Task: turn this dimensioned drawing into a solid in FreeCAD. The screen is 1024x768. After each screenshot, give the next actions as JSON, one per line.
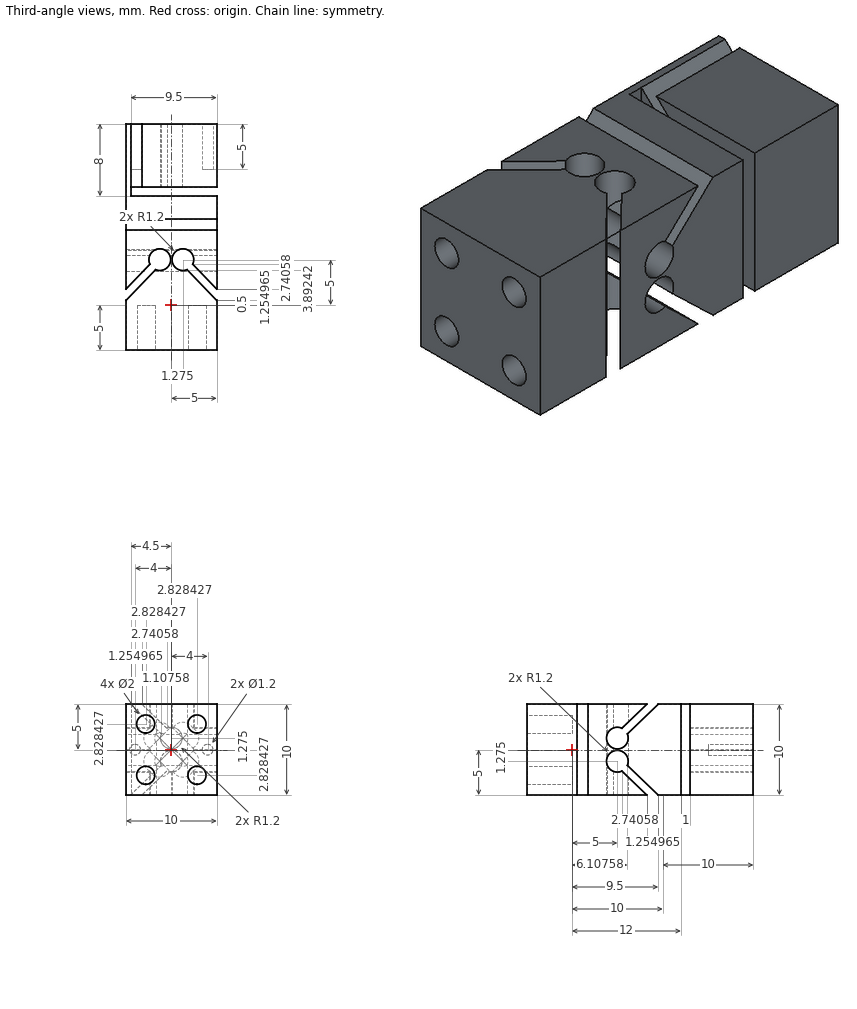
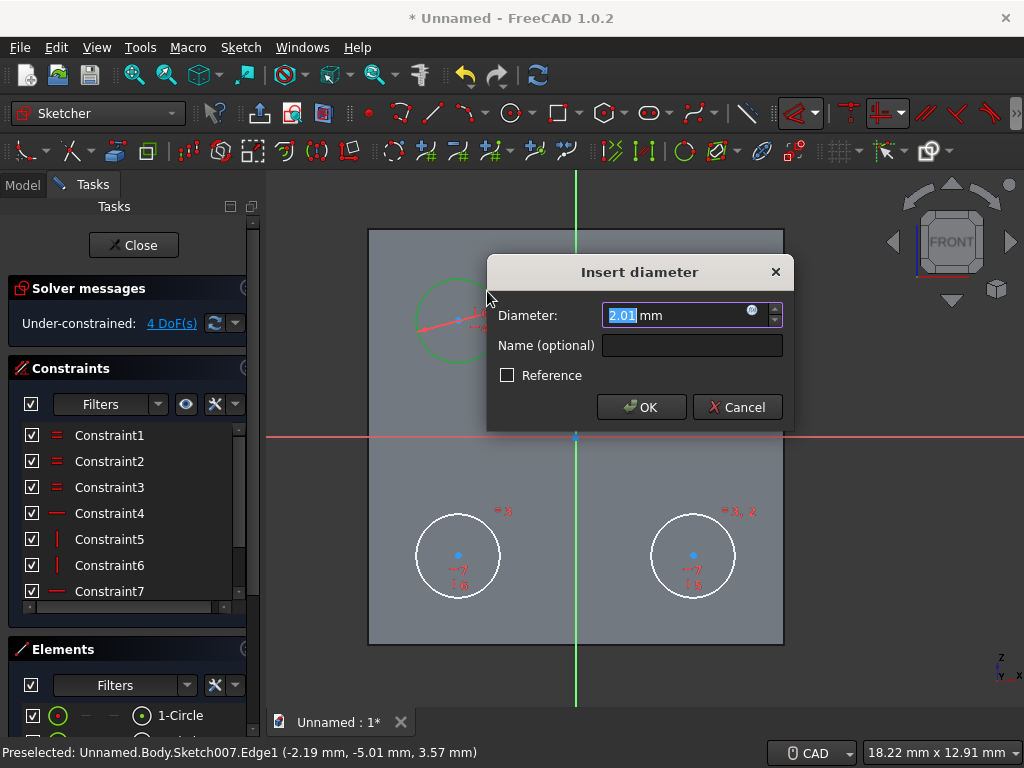
{"action": "type", "text": "2"}
{"action": "key", "text": "Return"}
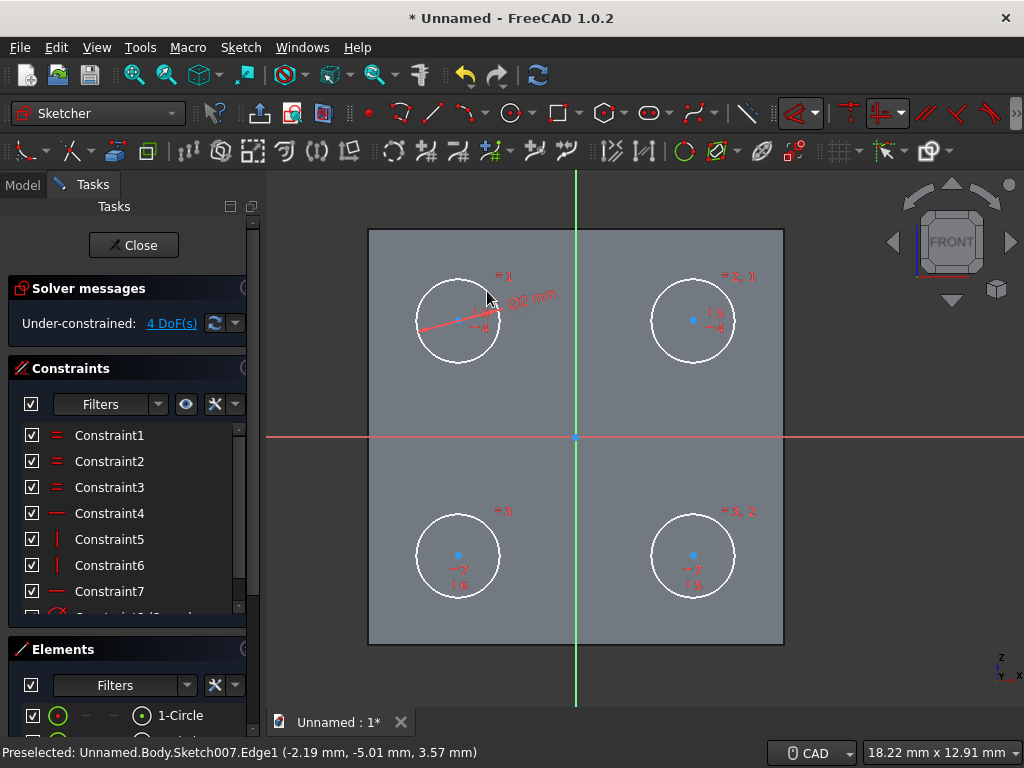
{"action": "left_click", "coordinate": [458, 321]}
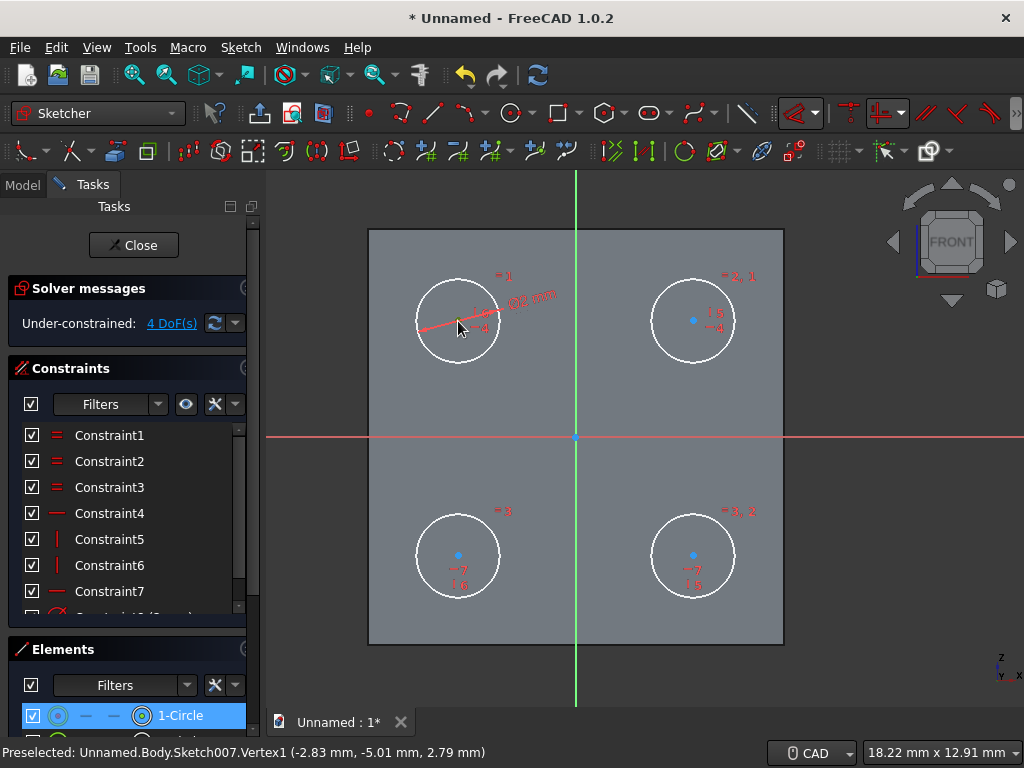
{"action": "key", "text": "l"}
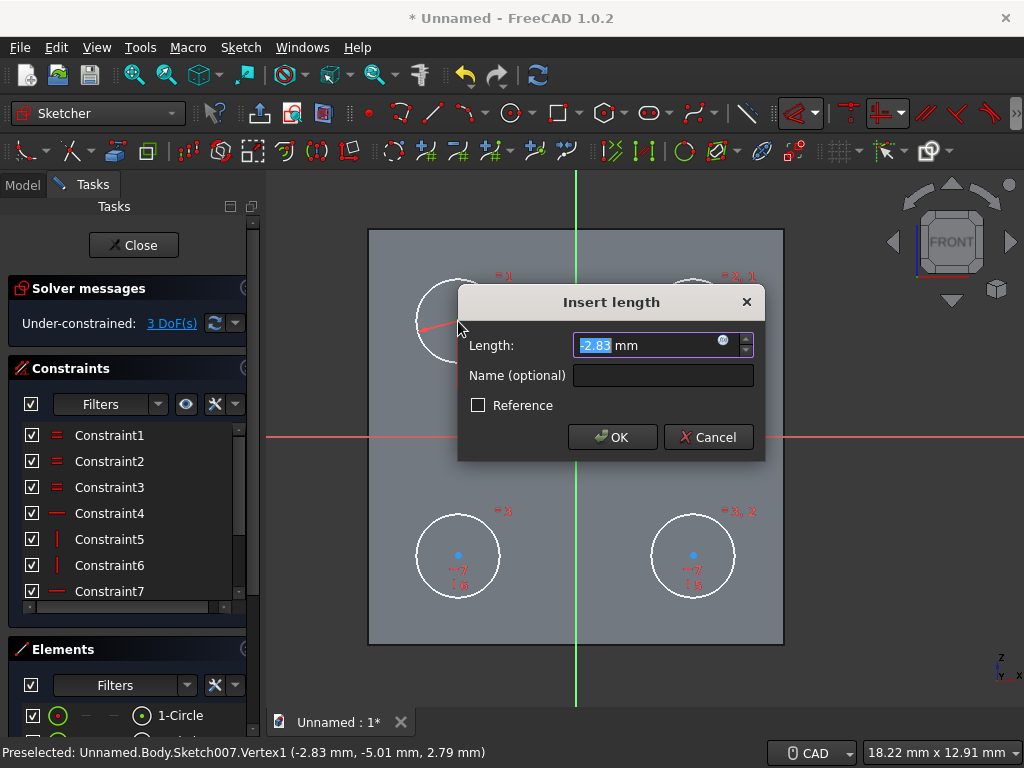
{"action": "type", "text": "-2.828427"}
{"action": "key", "text": "Return"}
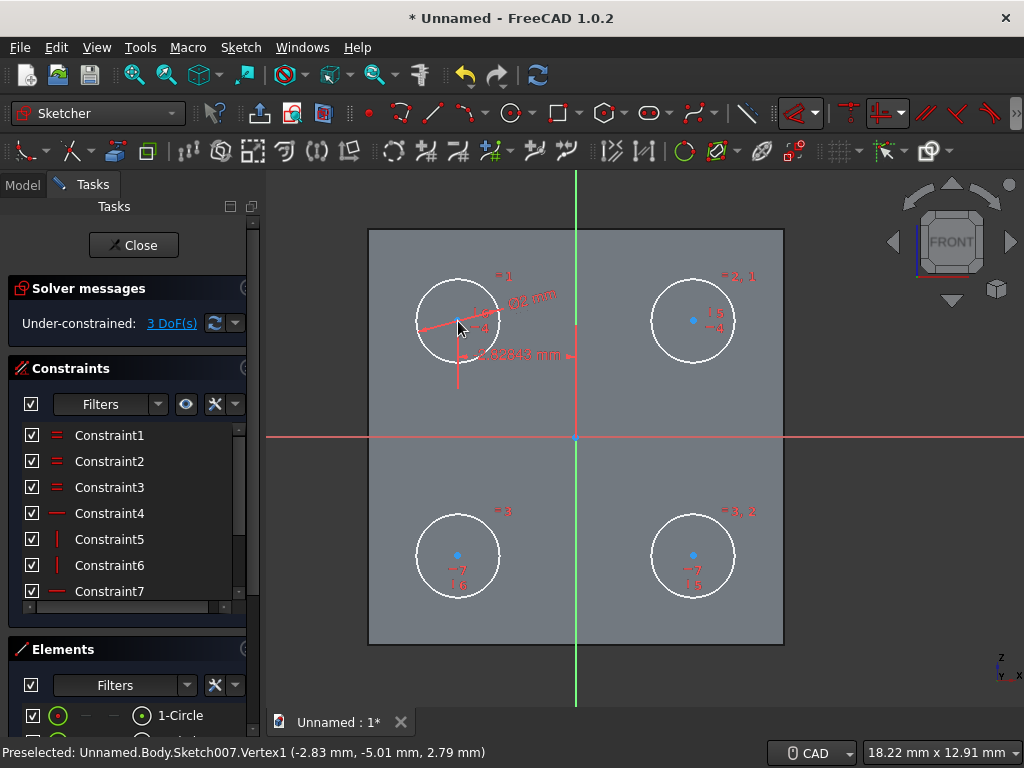
{"action": "left_click", "coordinate": [458, 321]}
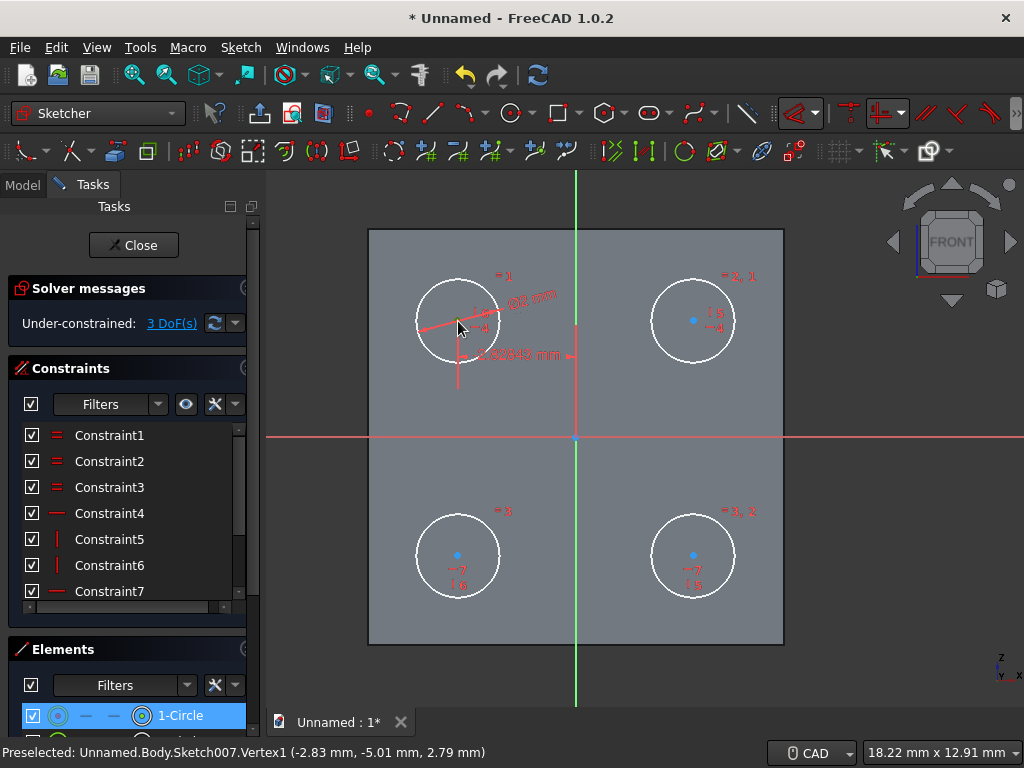
{"action": "key", "text": "i"}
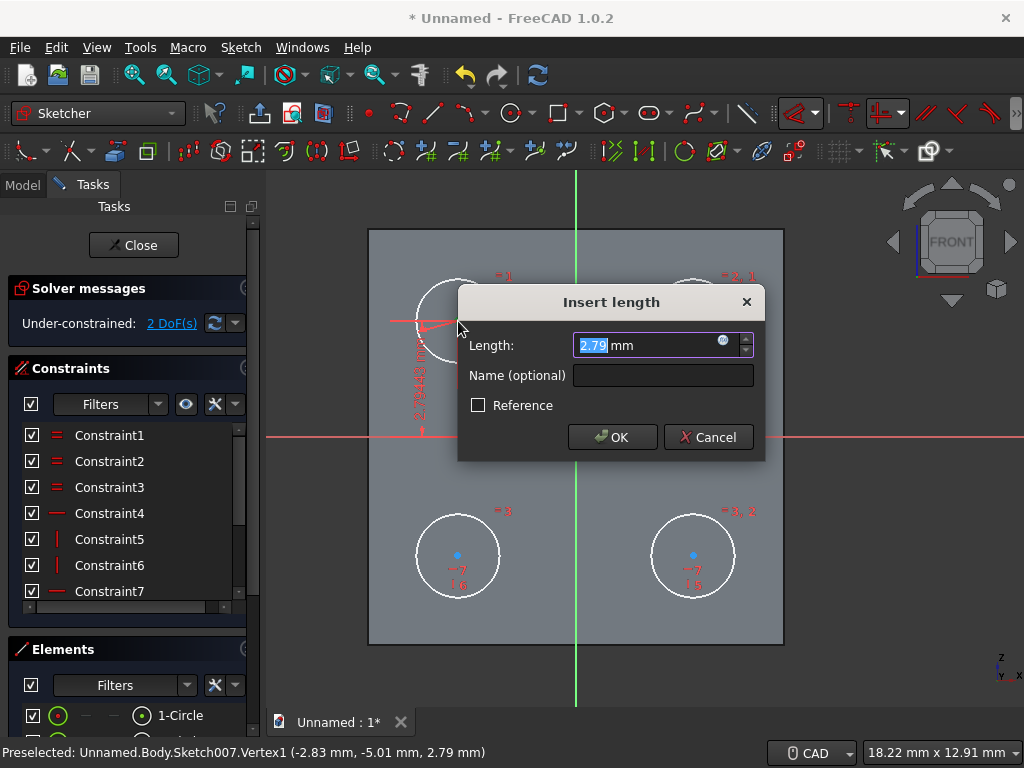
{"action": "type", "text": "2.828427"}
{"action": "key", "text": "Return"}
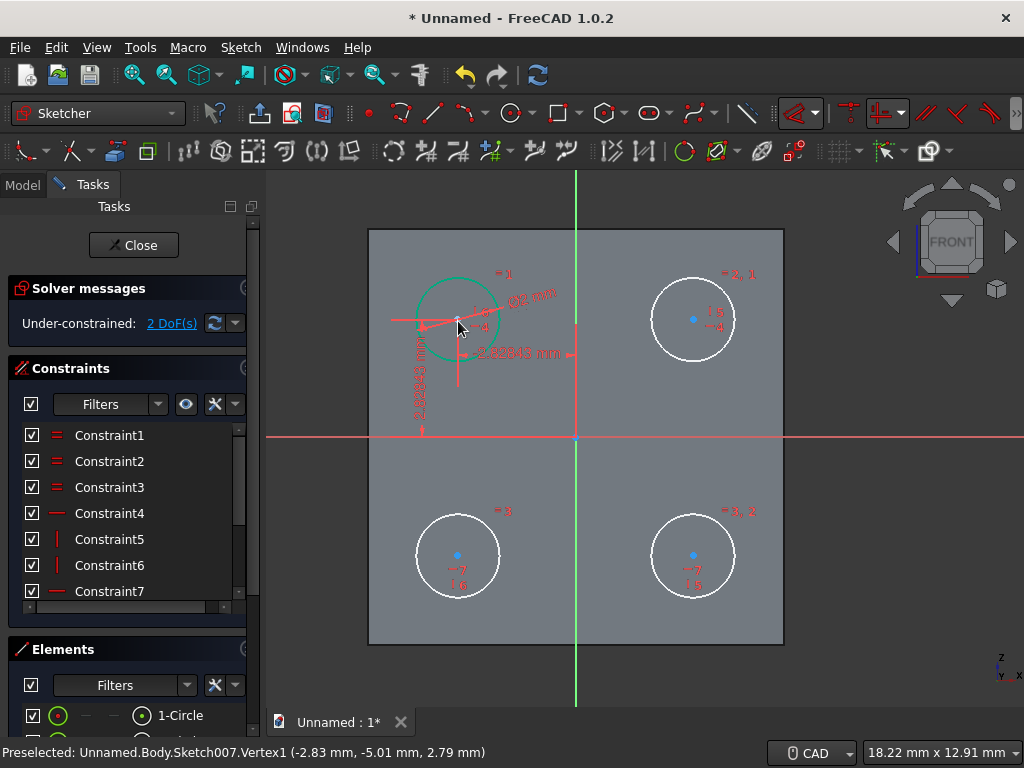
{"action": "left_click", "coordinate": [693, 320]}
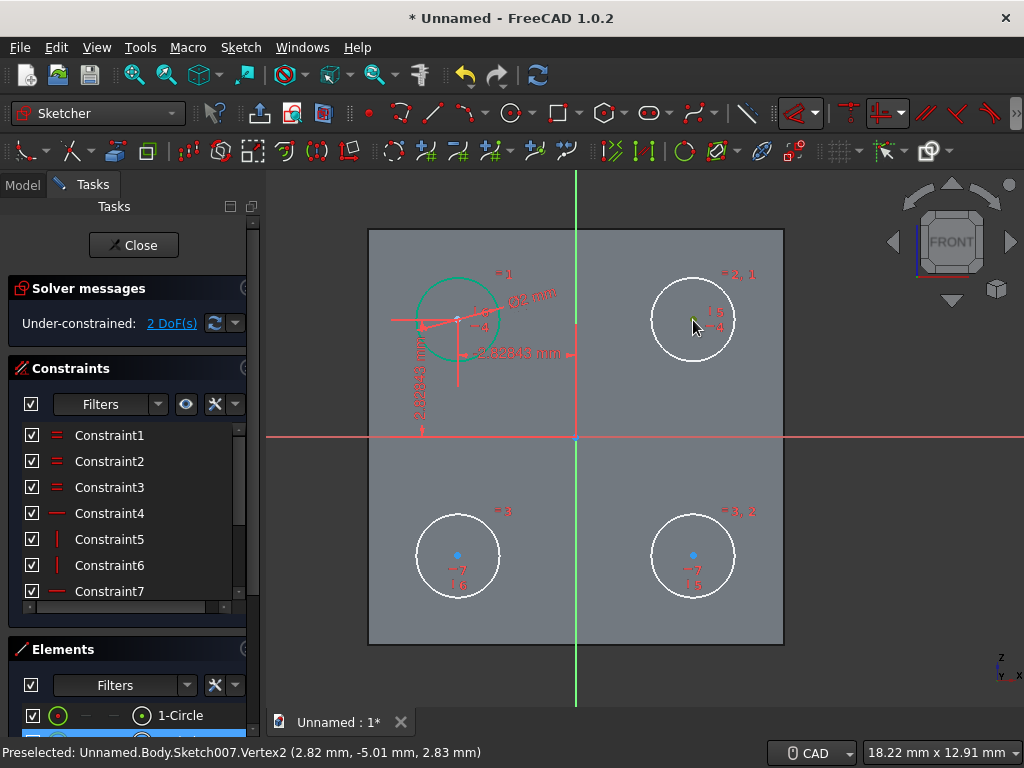
{"action": "left_click", "coordinate": [818, 114]}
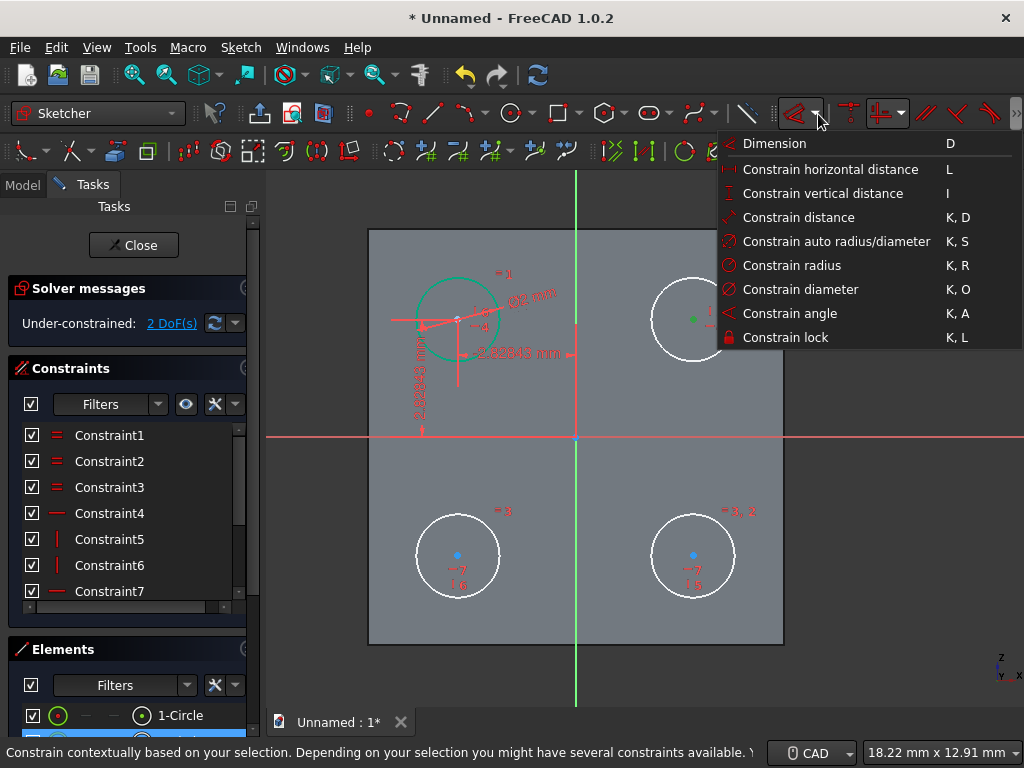
{"action": "left_click", "coordinate": [870, 169]}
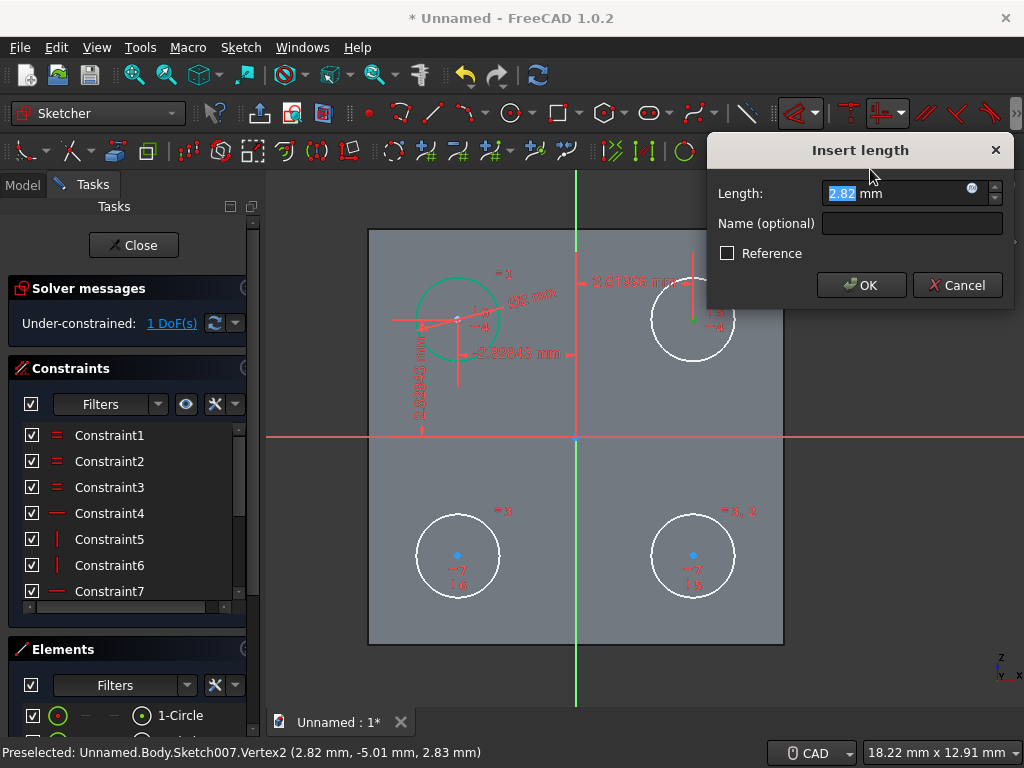
{"action": "type", "text": "2.828427"}
{"action": "key", "text": "Return"}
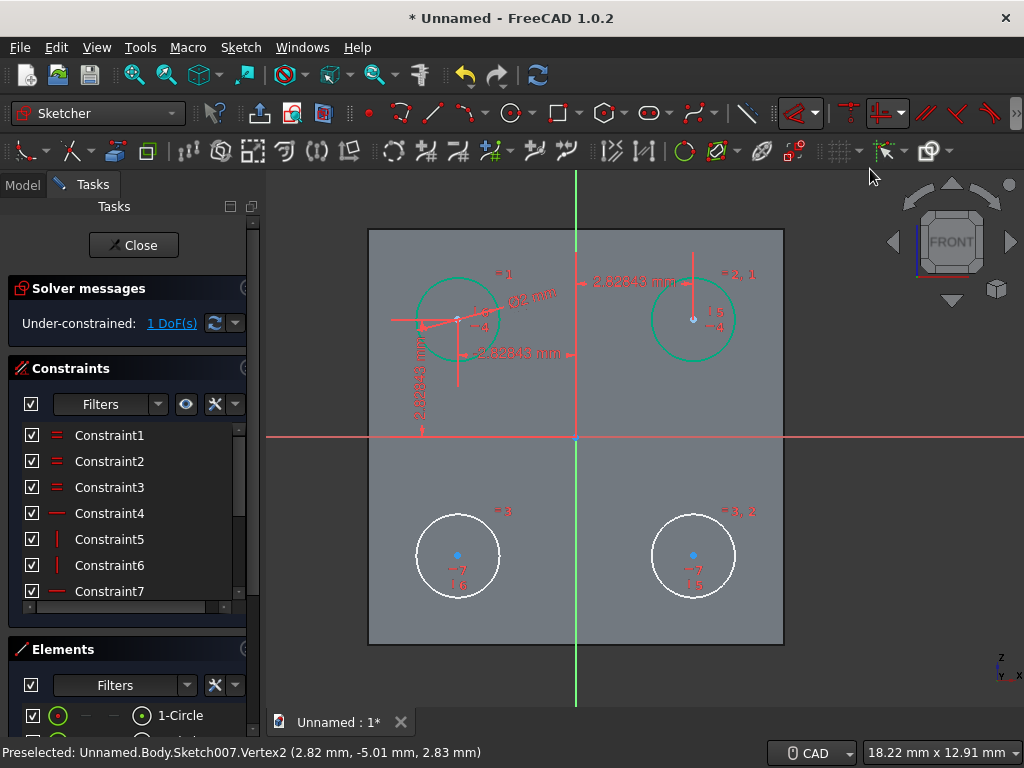
{"action": "left_click", "coordinate": [693, 556]}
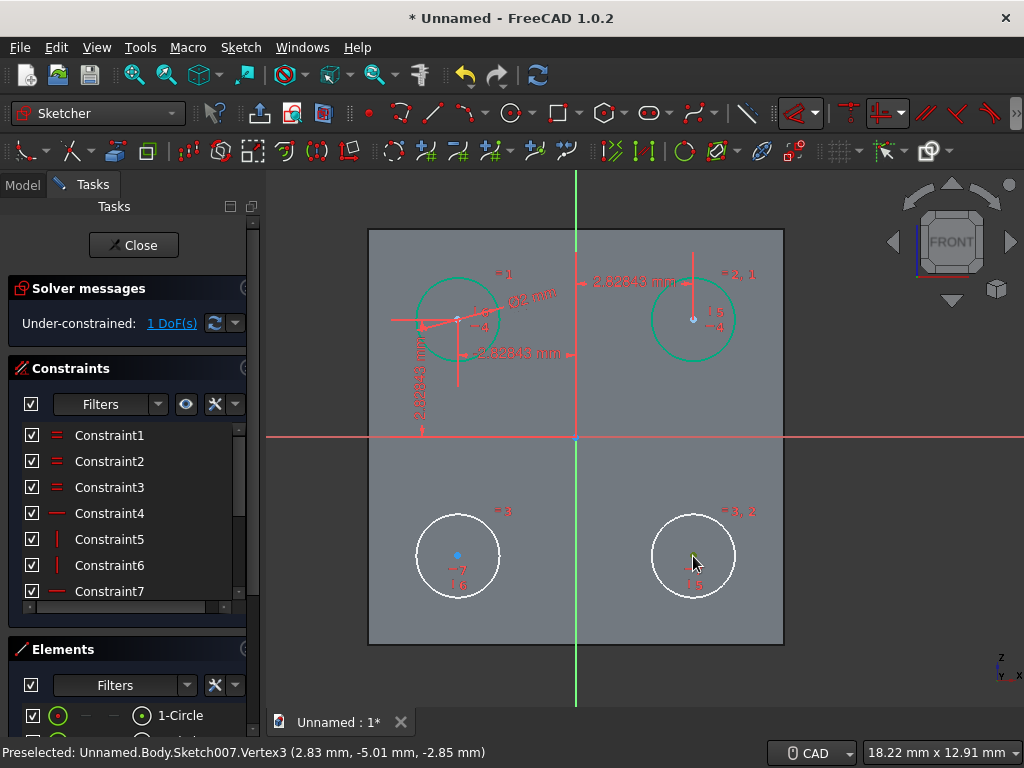
{"action": "key", "text": "i"}